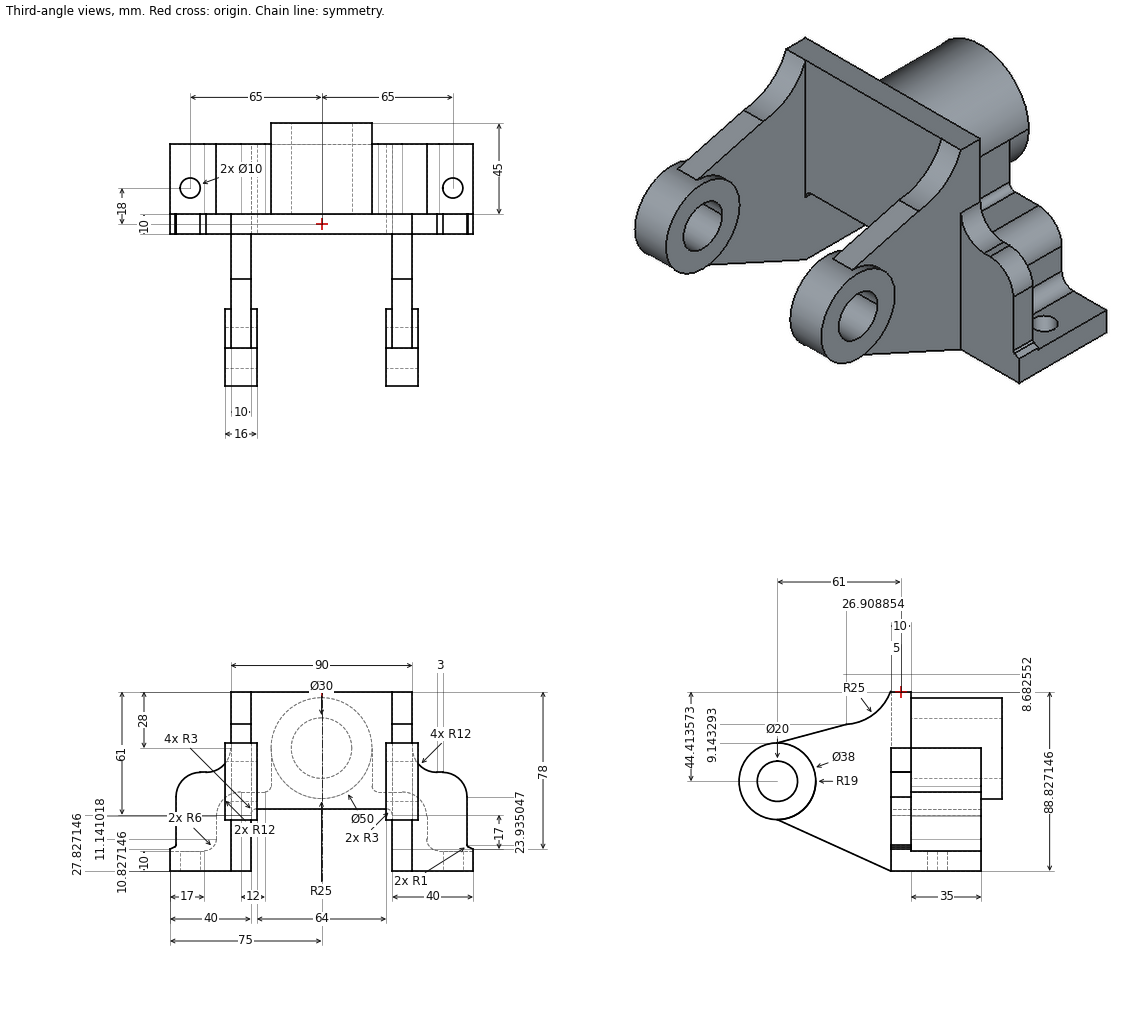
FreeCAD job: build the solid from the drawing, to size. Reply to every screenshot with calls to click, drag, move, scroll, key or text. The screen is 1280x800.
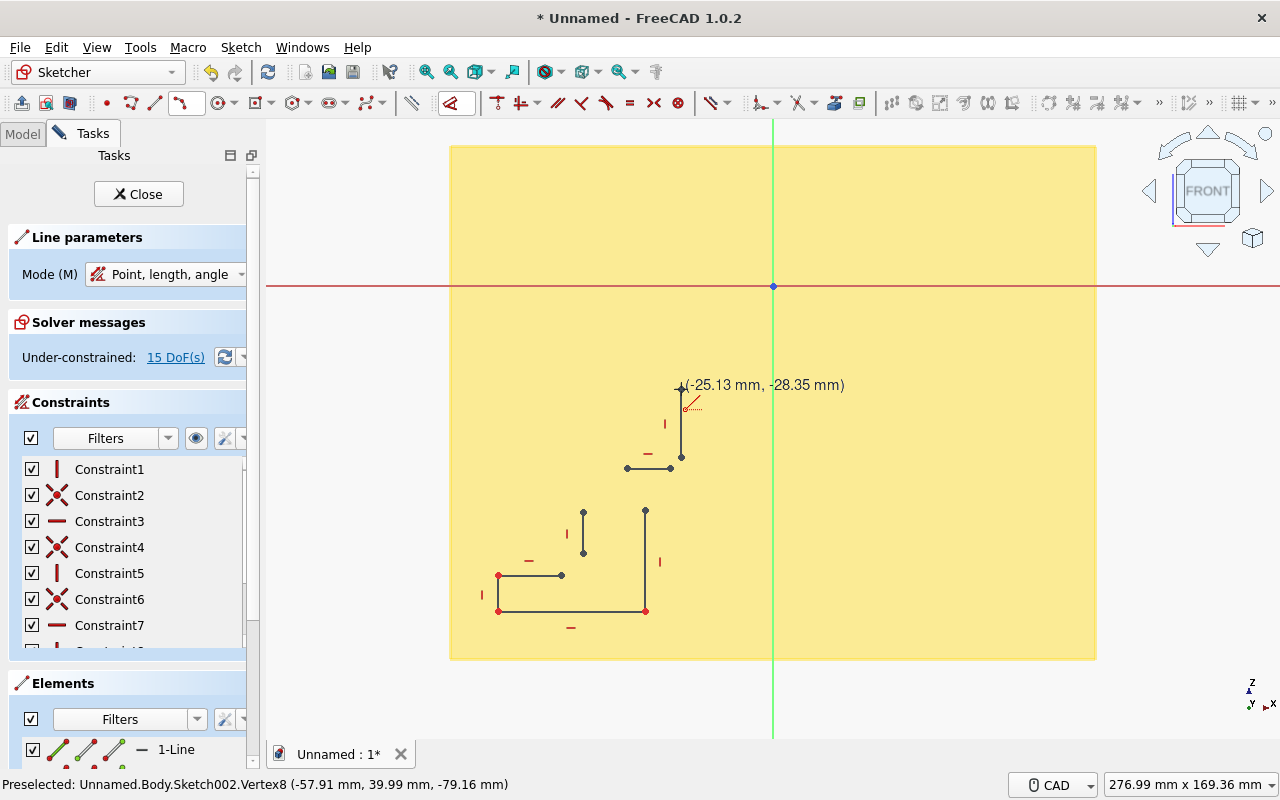
click(865, 389)
click(865, 457)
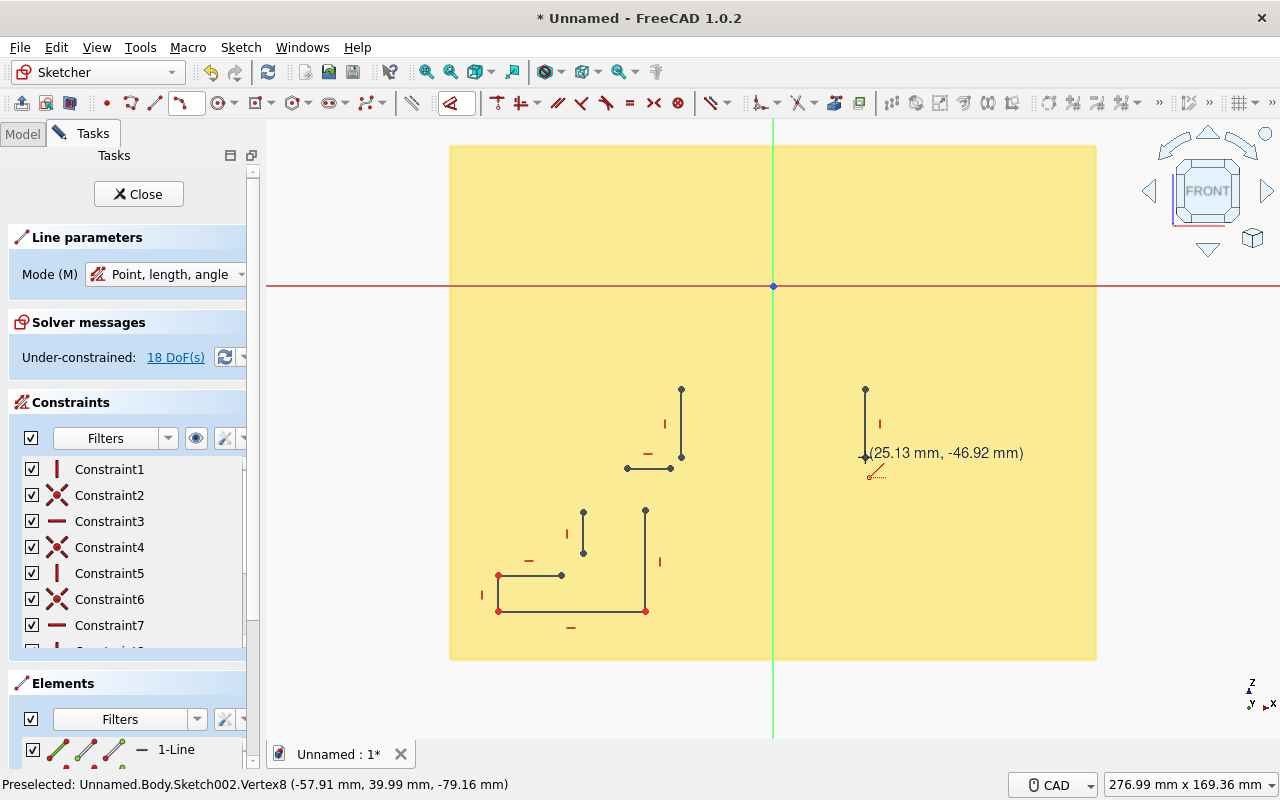
click(876, 468)
click(919, 468)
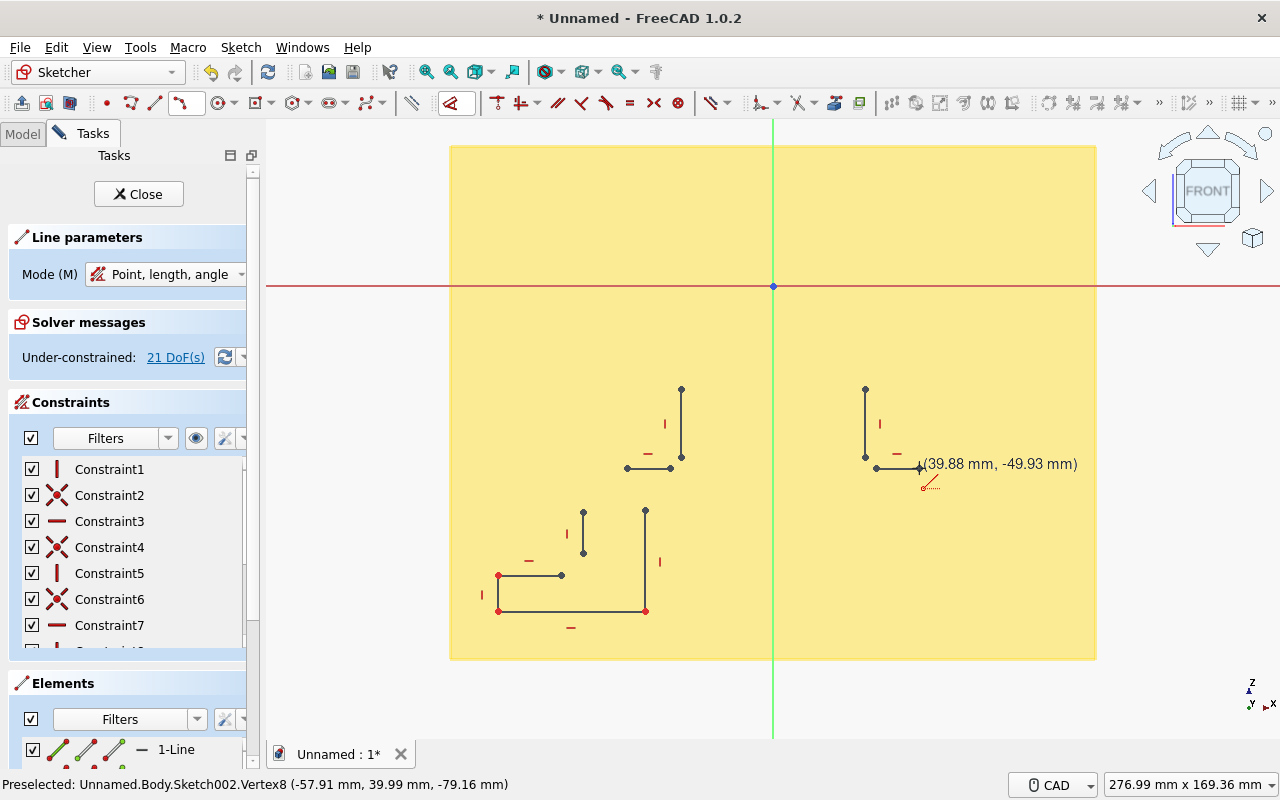
click(963, 512)
click(963, 553)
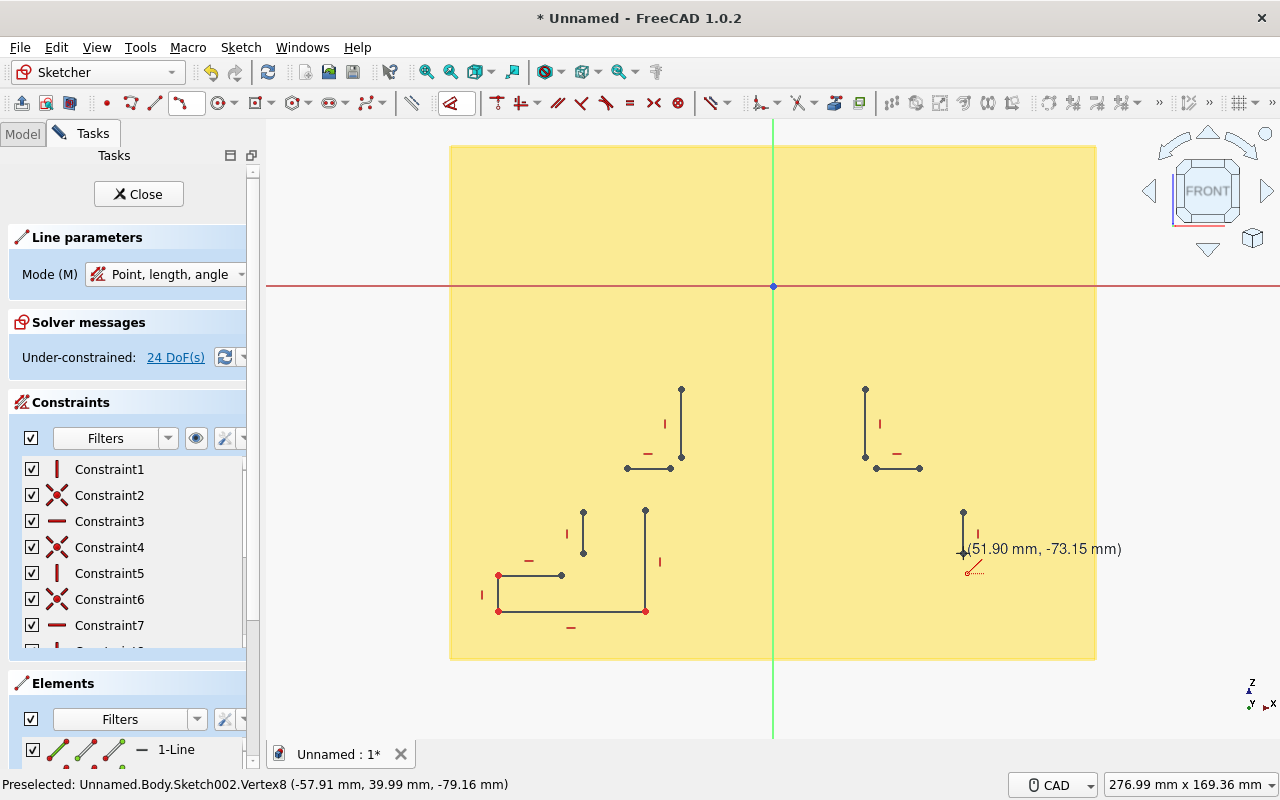
key(g)
key(m)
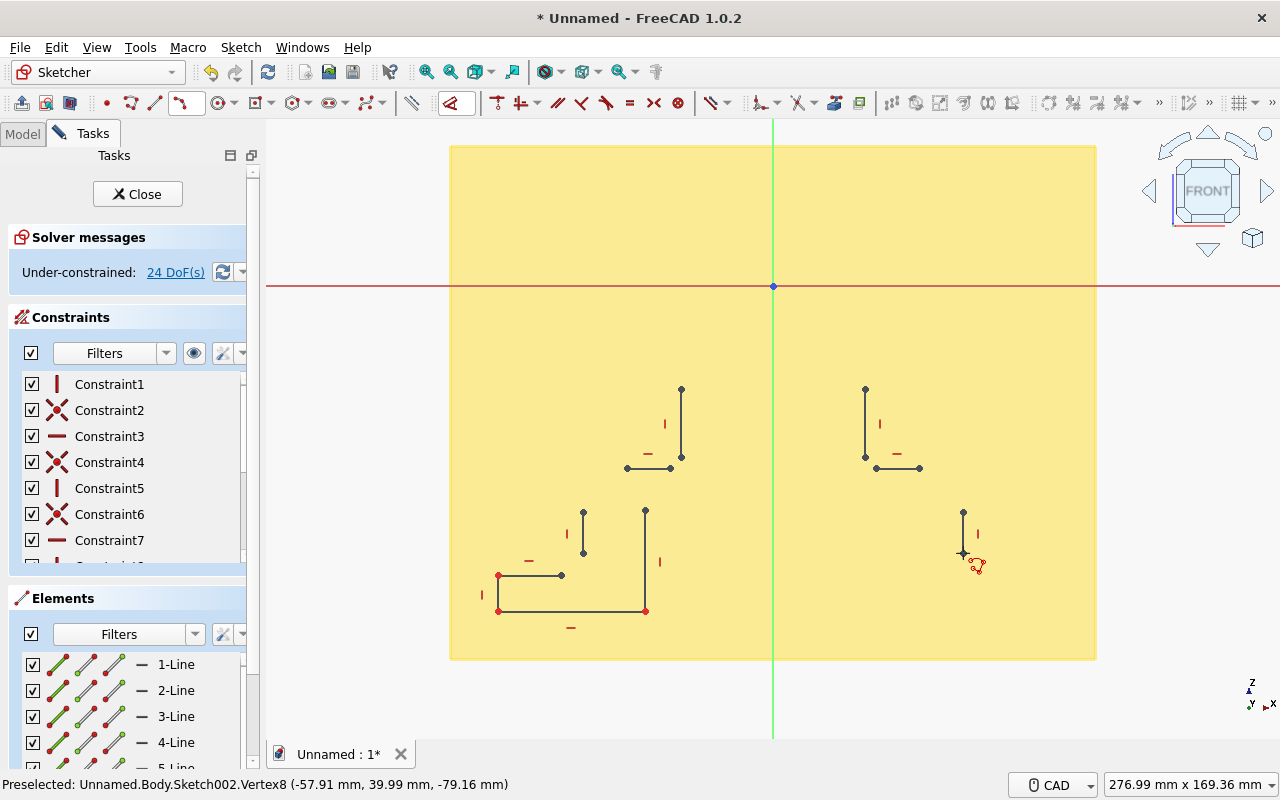
click(985, 575)
click(1048, 575)
click(1048, 611)
click(901, 611)
click(901, 510)
right_click(901, 510)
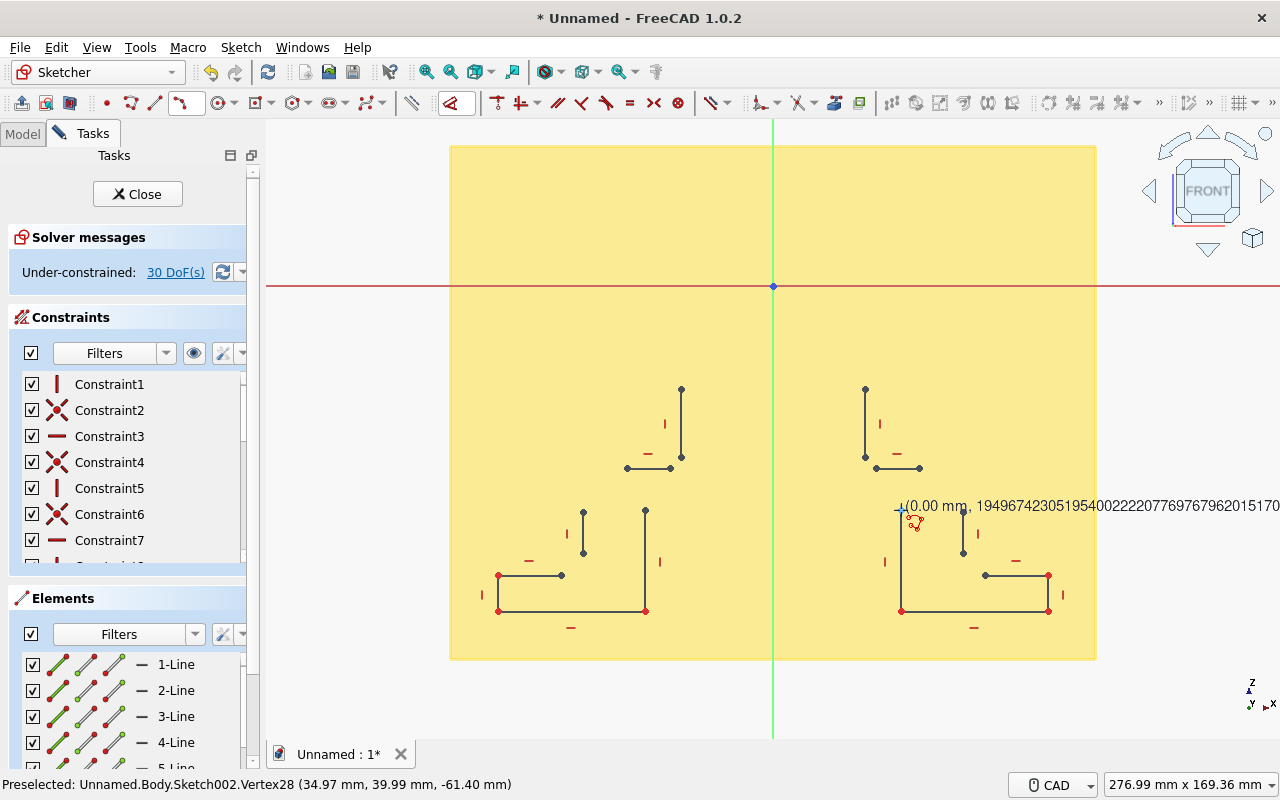
key(g)
key(l)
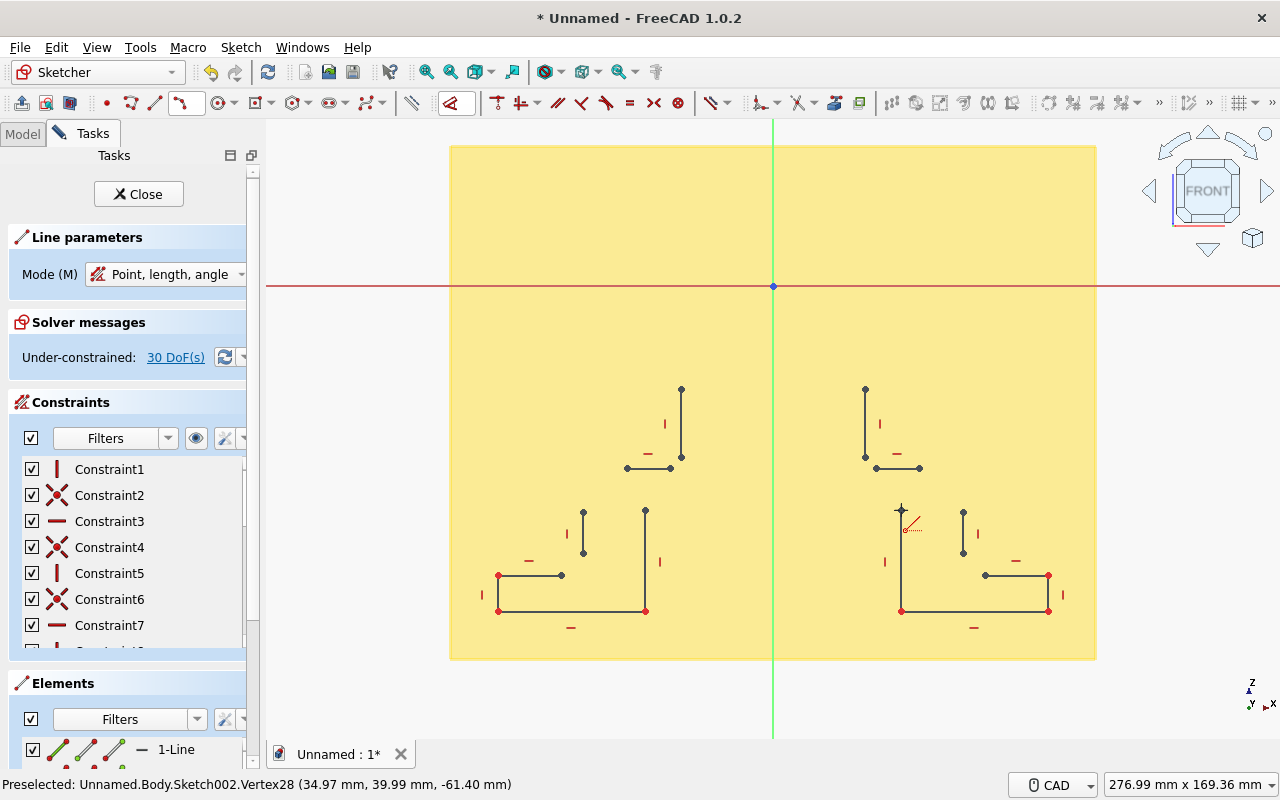
click(890, 499)
click(656, 499)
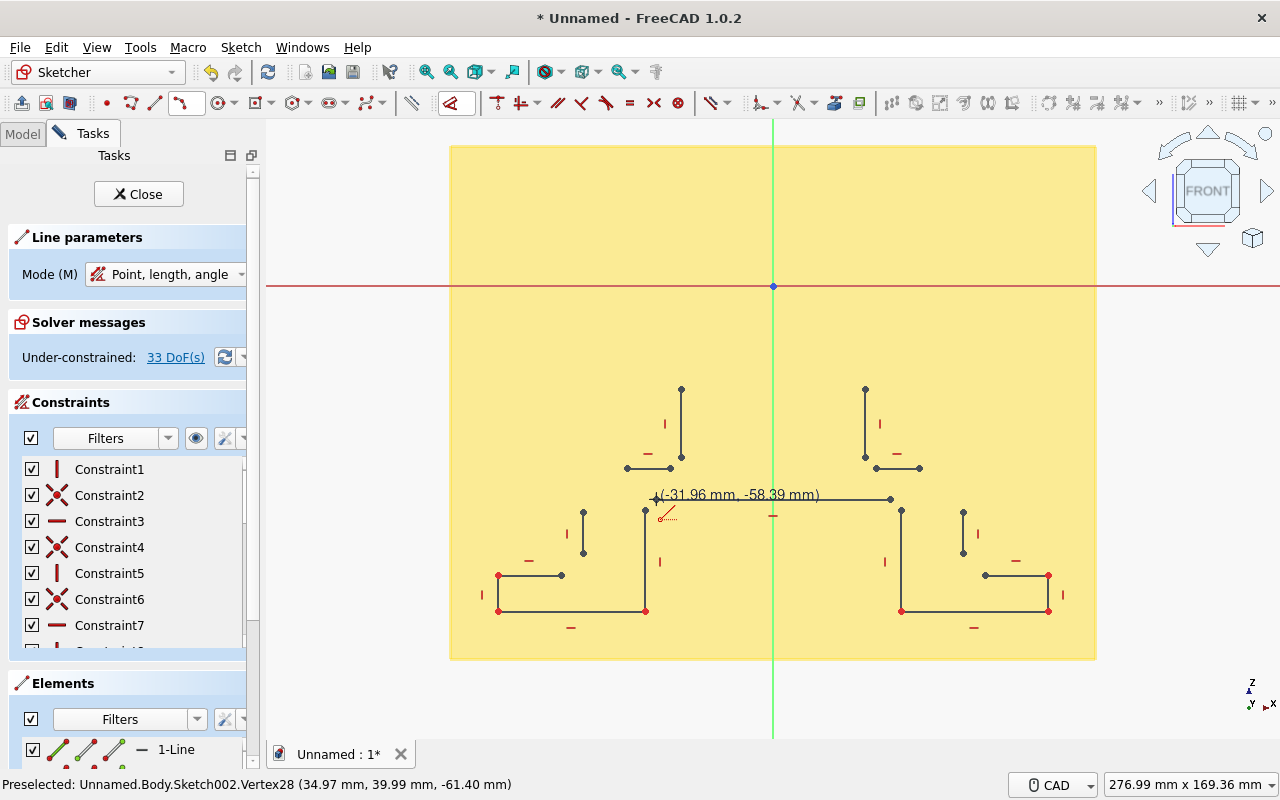
key(g)
key(3)
key(a)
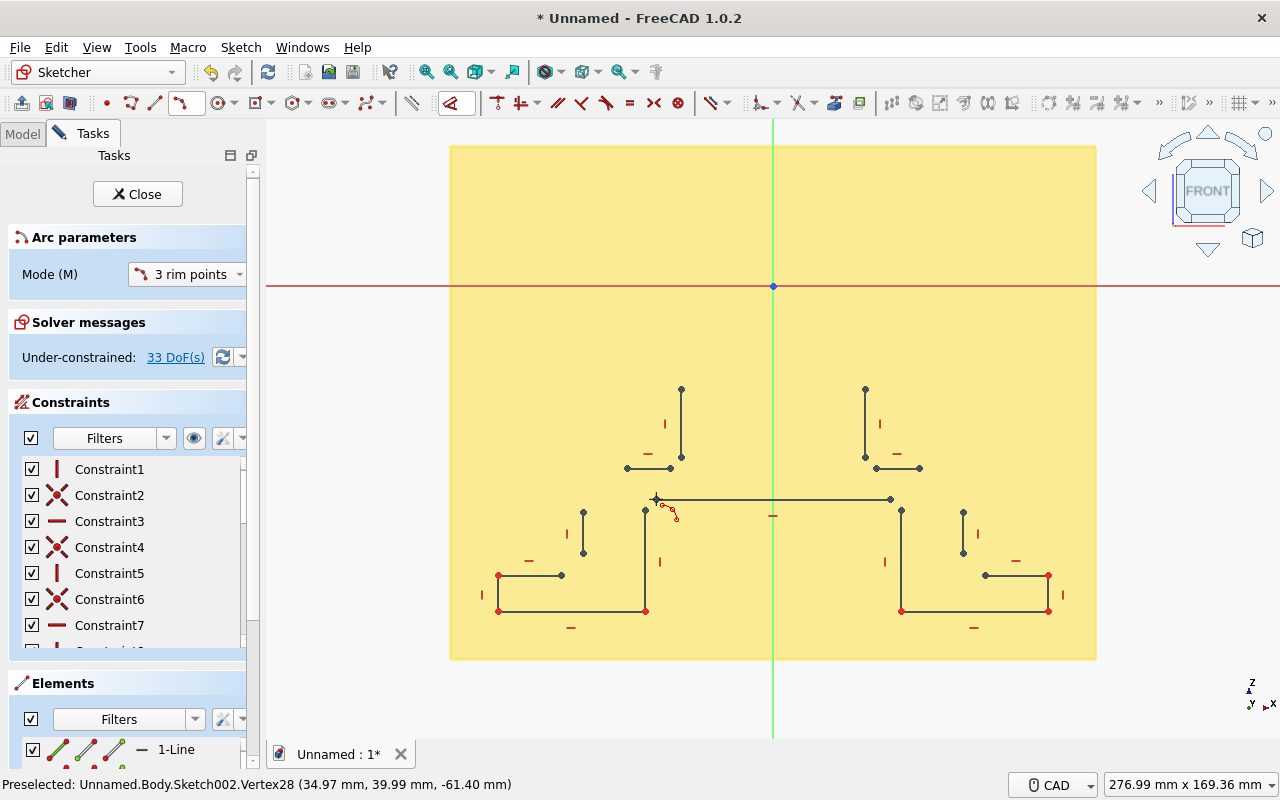
click(561, 576)
click(583, 554)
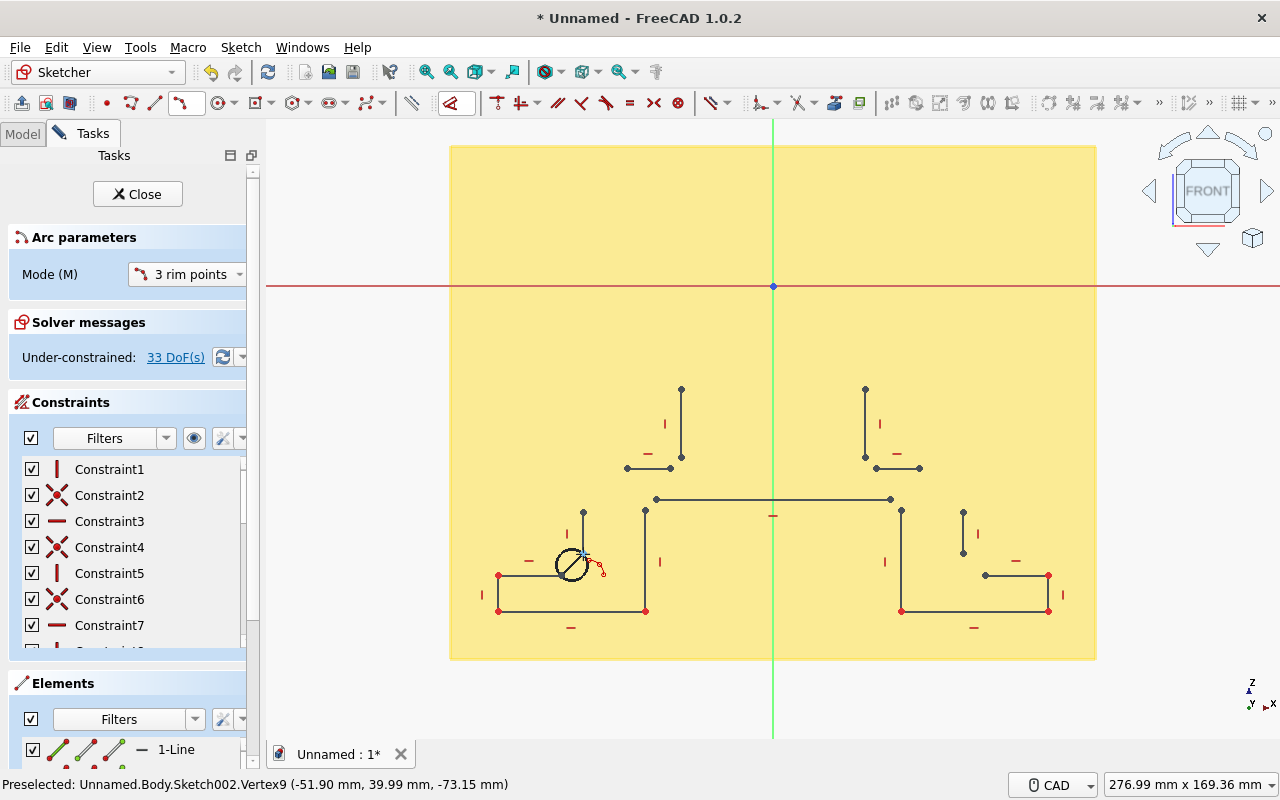
scroll(576, 568, up, 5)